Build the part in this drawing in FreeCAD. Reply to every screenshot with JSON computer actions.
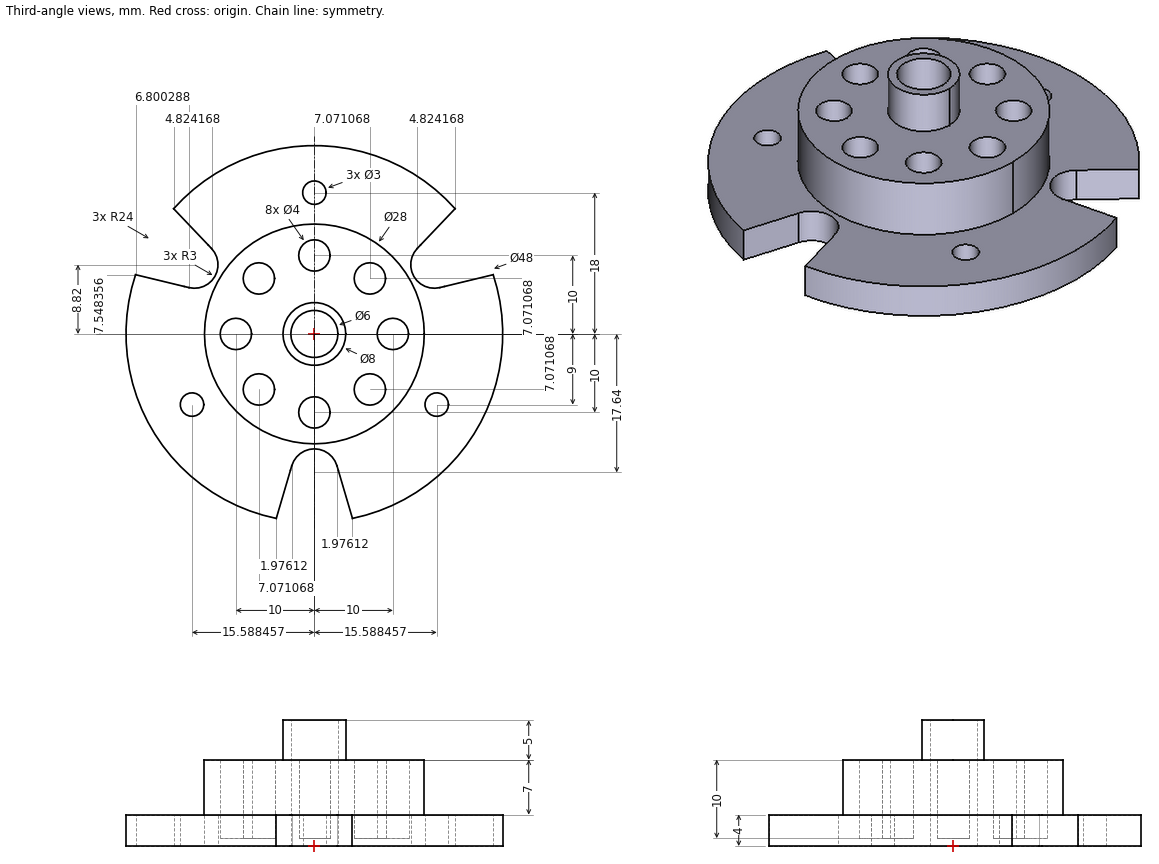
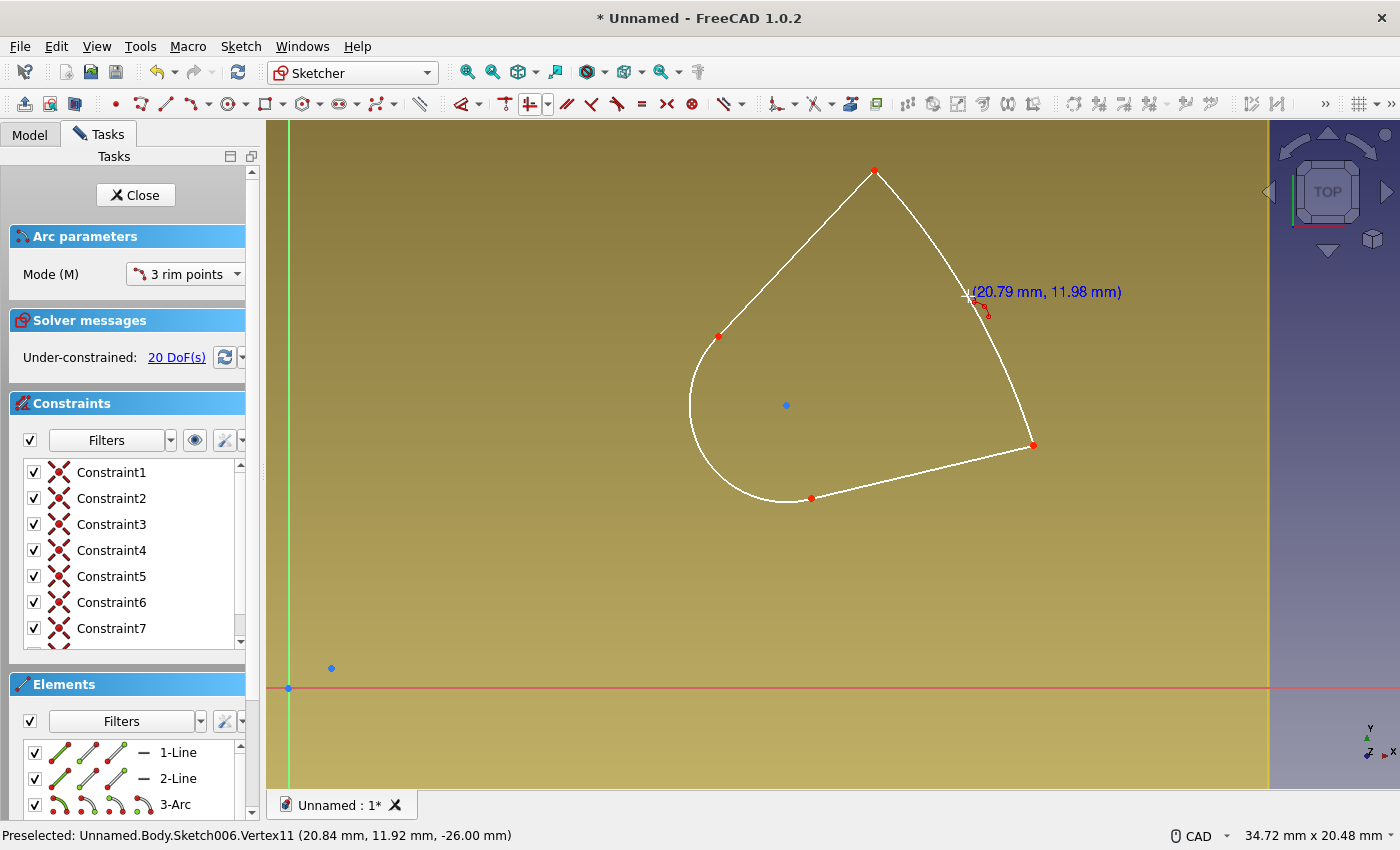
{"action": "key", "text": "g l"}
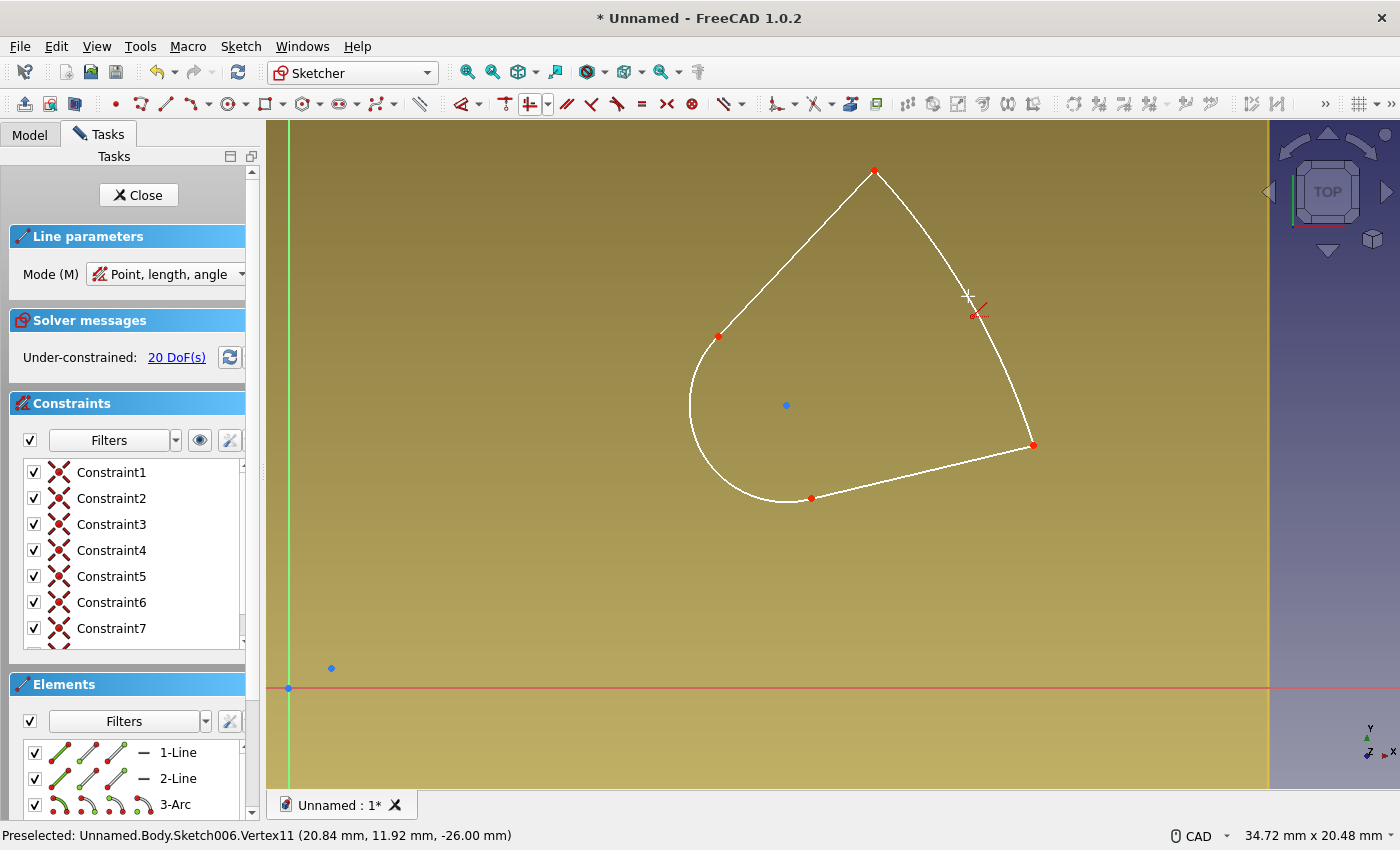
{"action": "scroll", "coordinate": [969, 297], "scroll_direction": "down", "scroll_amount": 6}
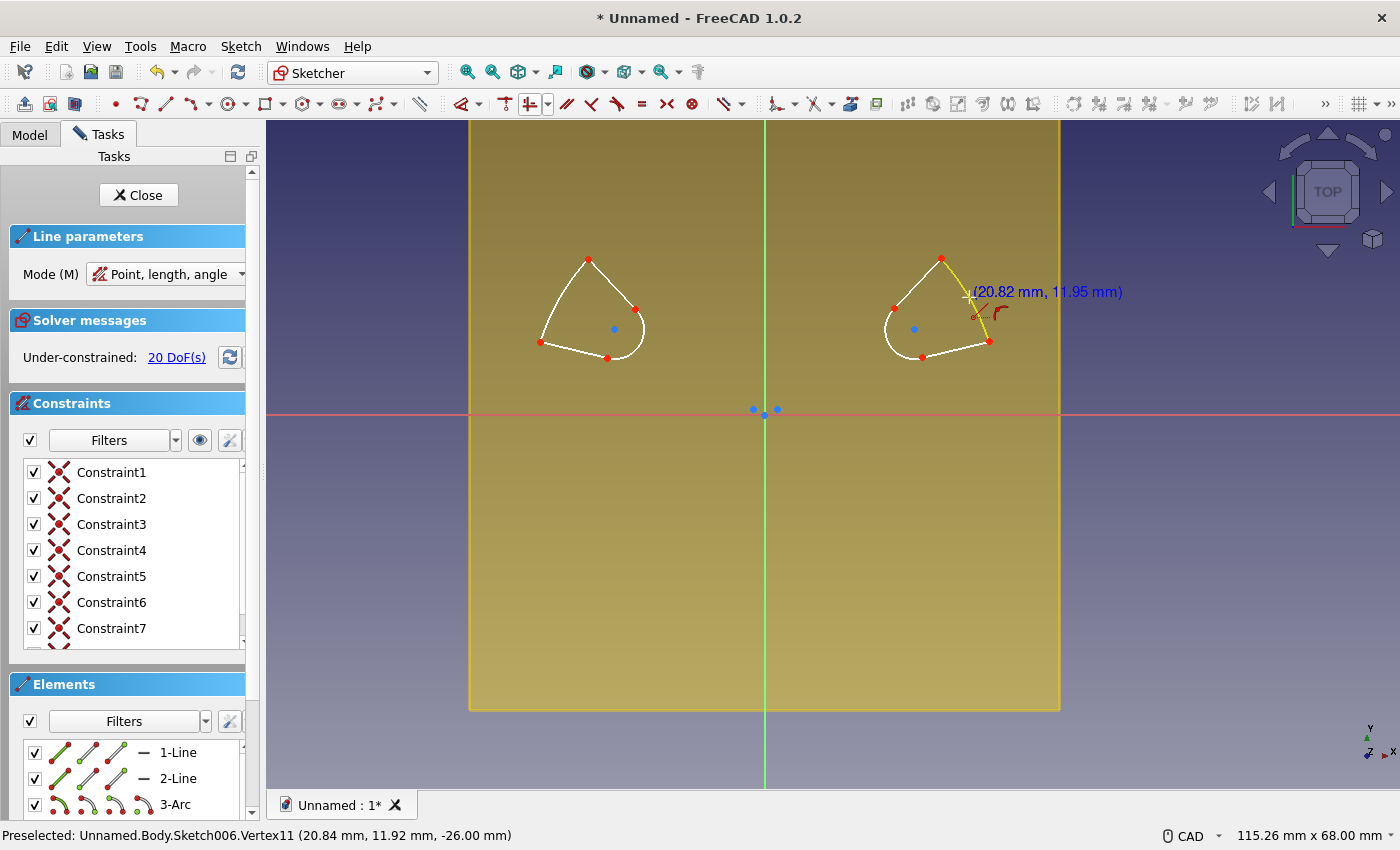
{"action": "left_click", "coordinate": [812, 646]}
{"action": "left_click", "coordinate": [793, 580]}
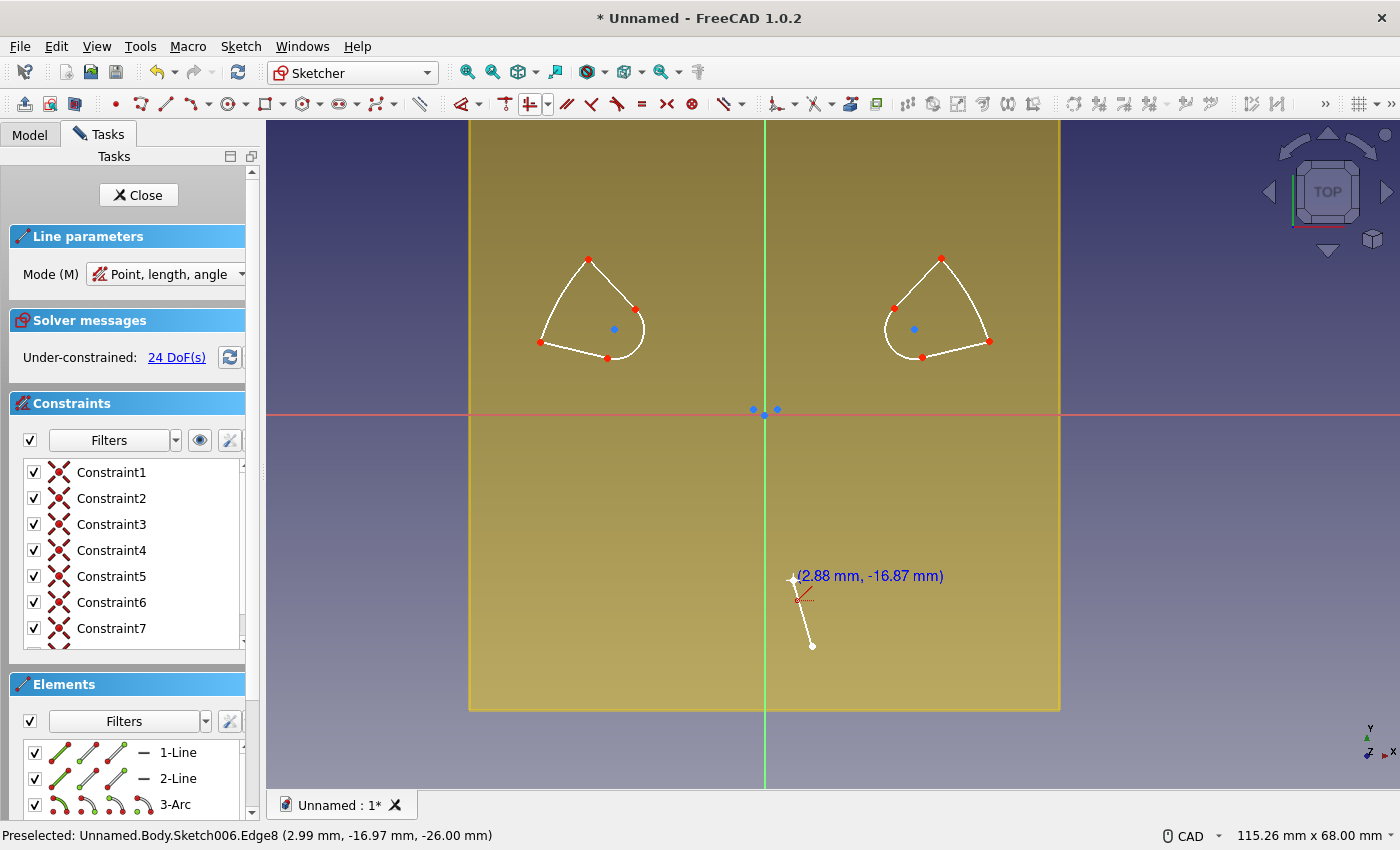
{"action": "left_click", "coordinate": [736, 580]}
{"action": "left_click", "coordinate": [717, 646]}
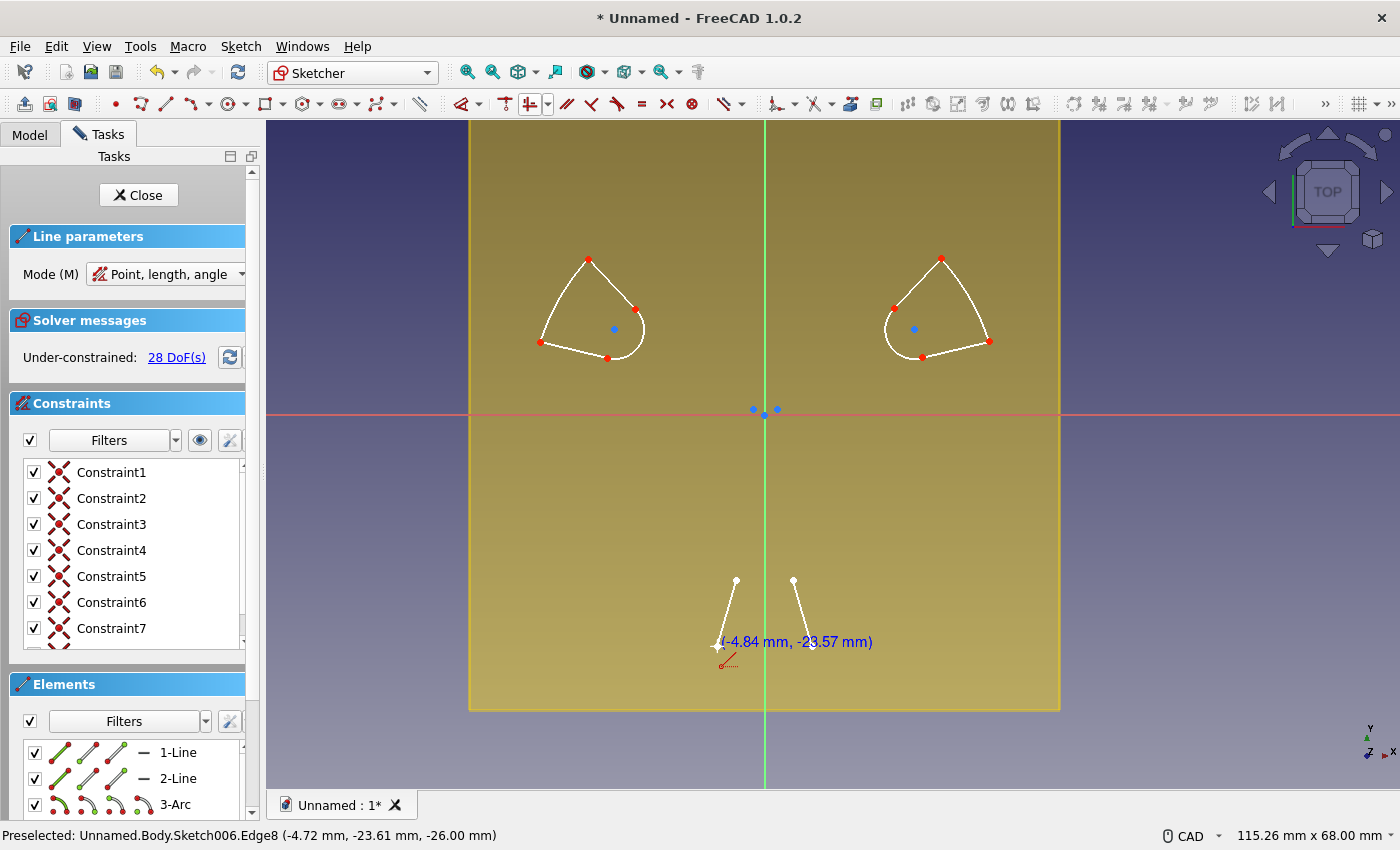
{"action": "left_click", "coordinate": [190, 104]}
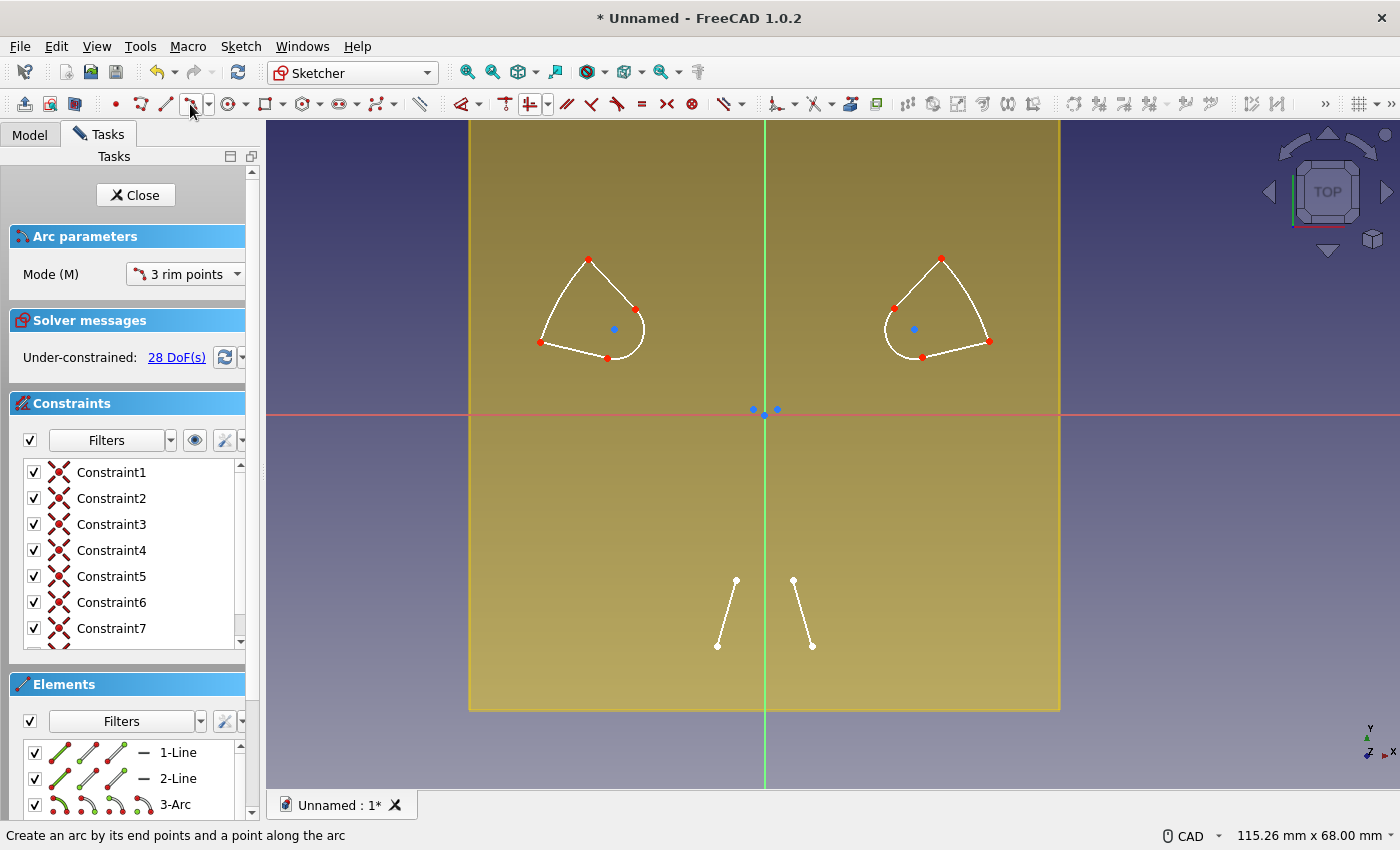
{"action": "left_click", "coordinate": [793, 581]}
{"action": "left_click", "coordinate": [736, 581]}
{"action": "left_click", "coordinate": [779, 563]}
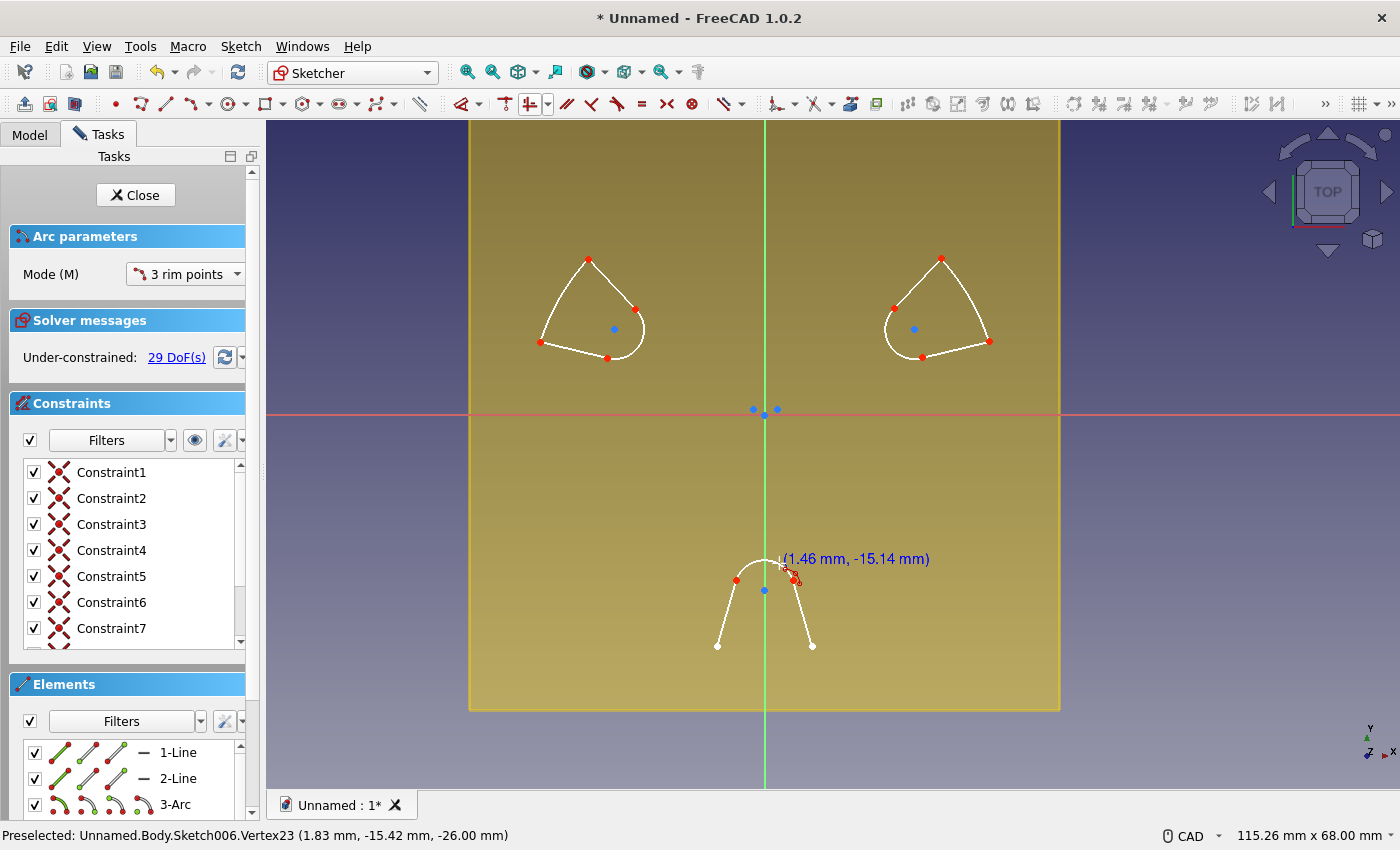
{"action": "left_click", "coordinate": [717, 647]}
{"action": "left_click", "coordinate": [812, 647]}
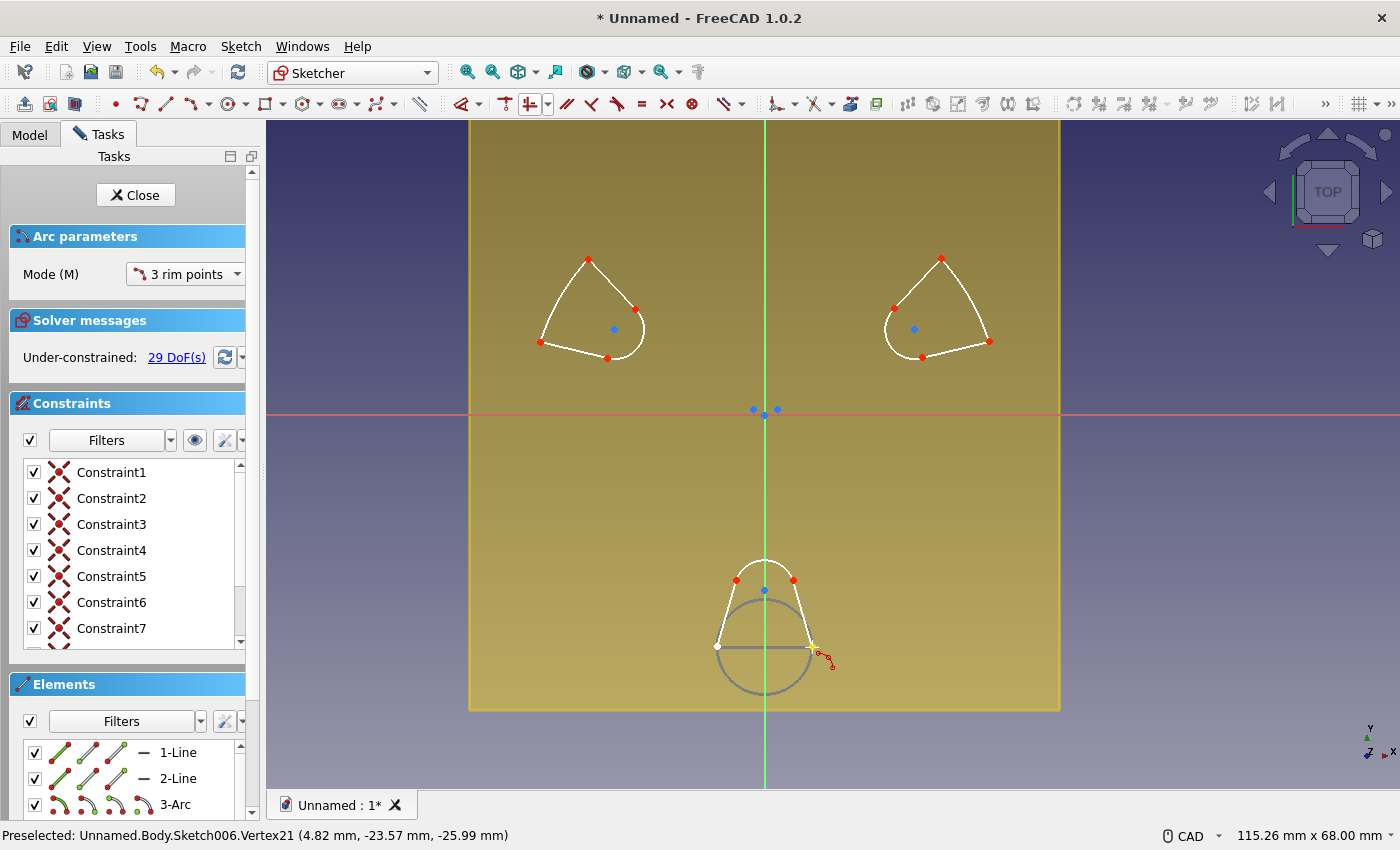
{"action": "scroll", "coordinate": [755, 651], "scroll_direction": "up", "scroll_amount": 7}